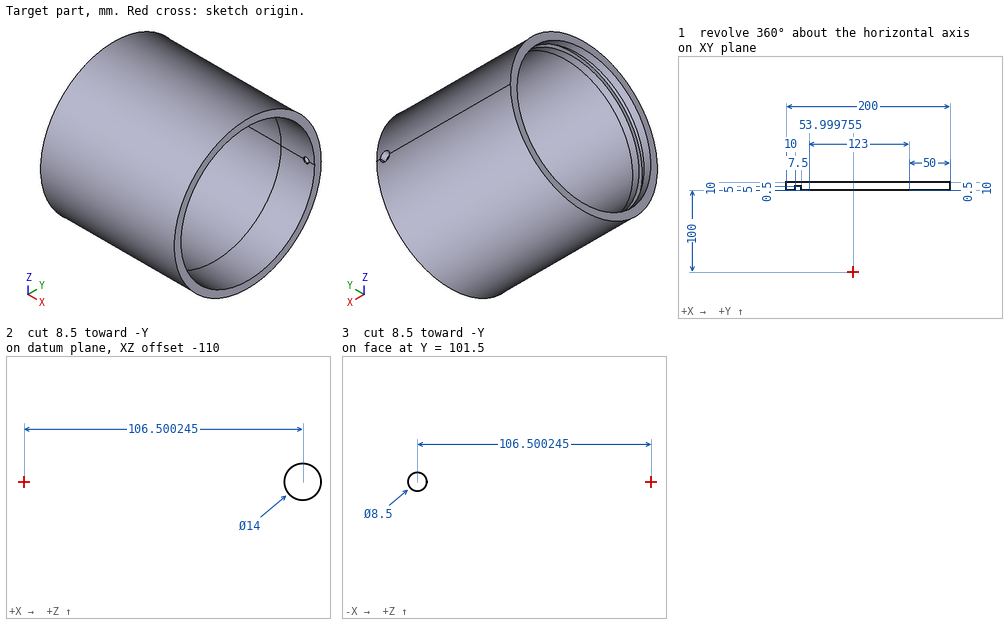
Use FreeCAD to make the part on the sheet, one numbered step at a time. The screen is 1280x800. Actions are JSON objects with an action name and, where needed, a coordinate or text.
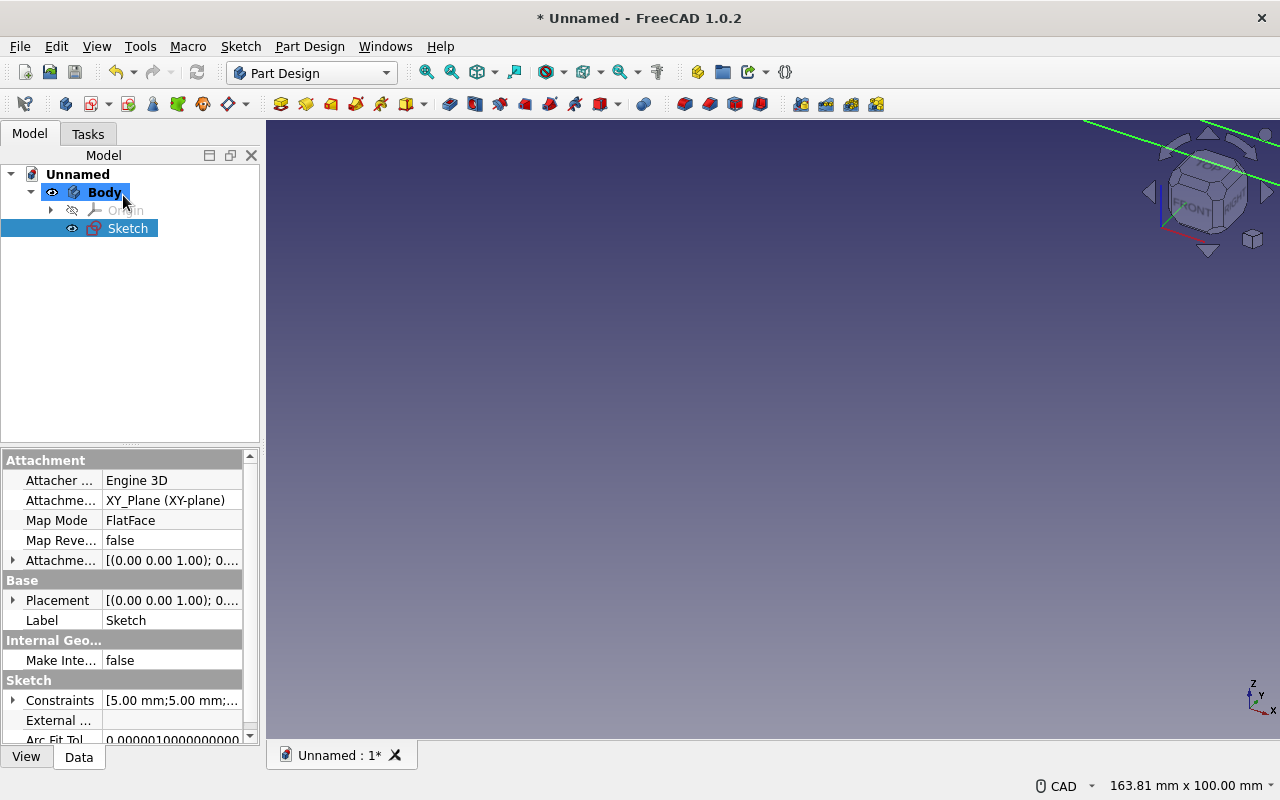
{"action": "left_click", "coordinate": [306, 104]}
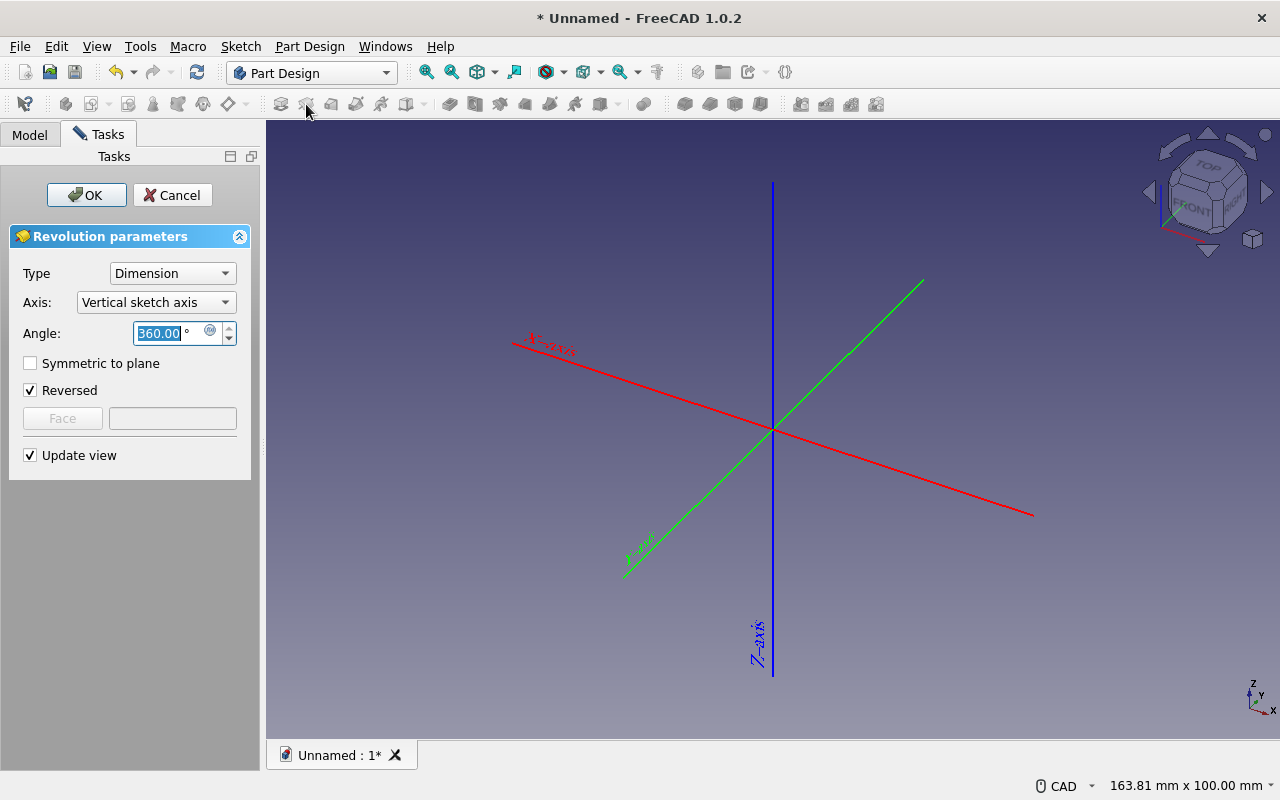
{"action": "left_click", "coordinate": [157, 302]}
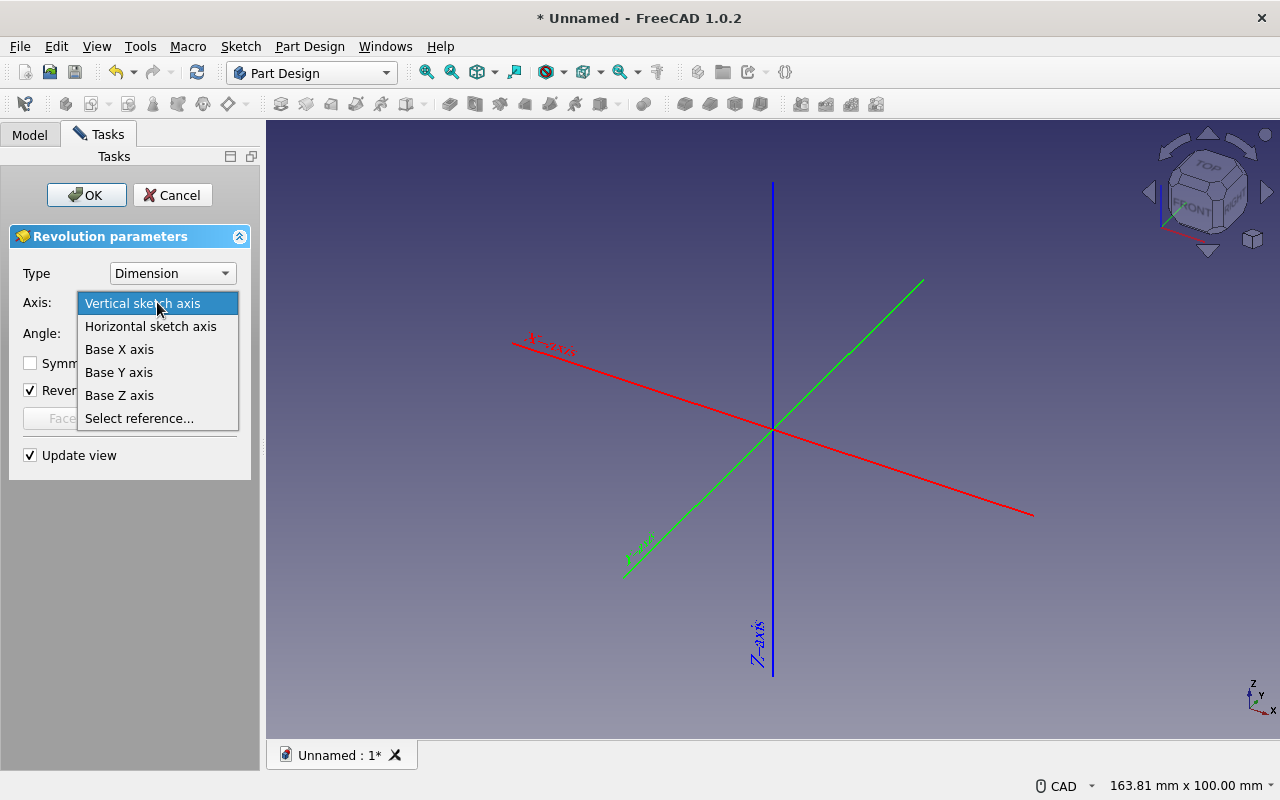
{"action": "left_click", "coordinate": [156, 326]}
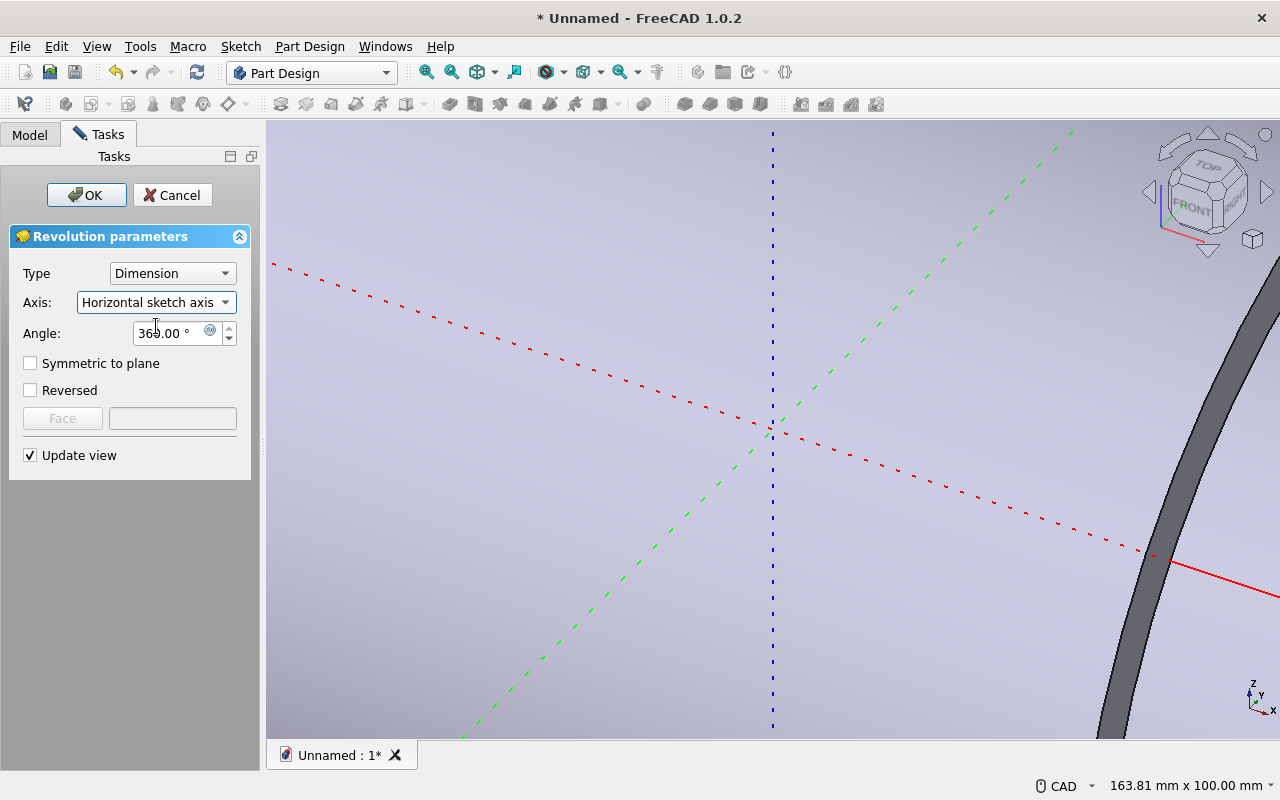
{"action": "left_click", "coordinate": [87, 195]}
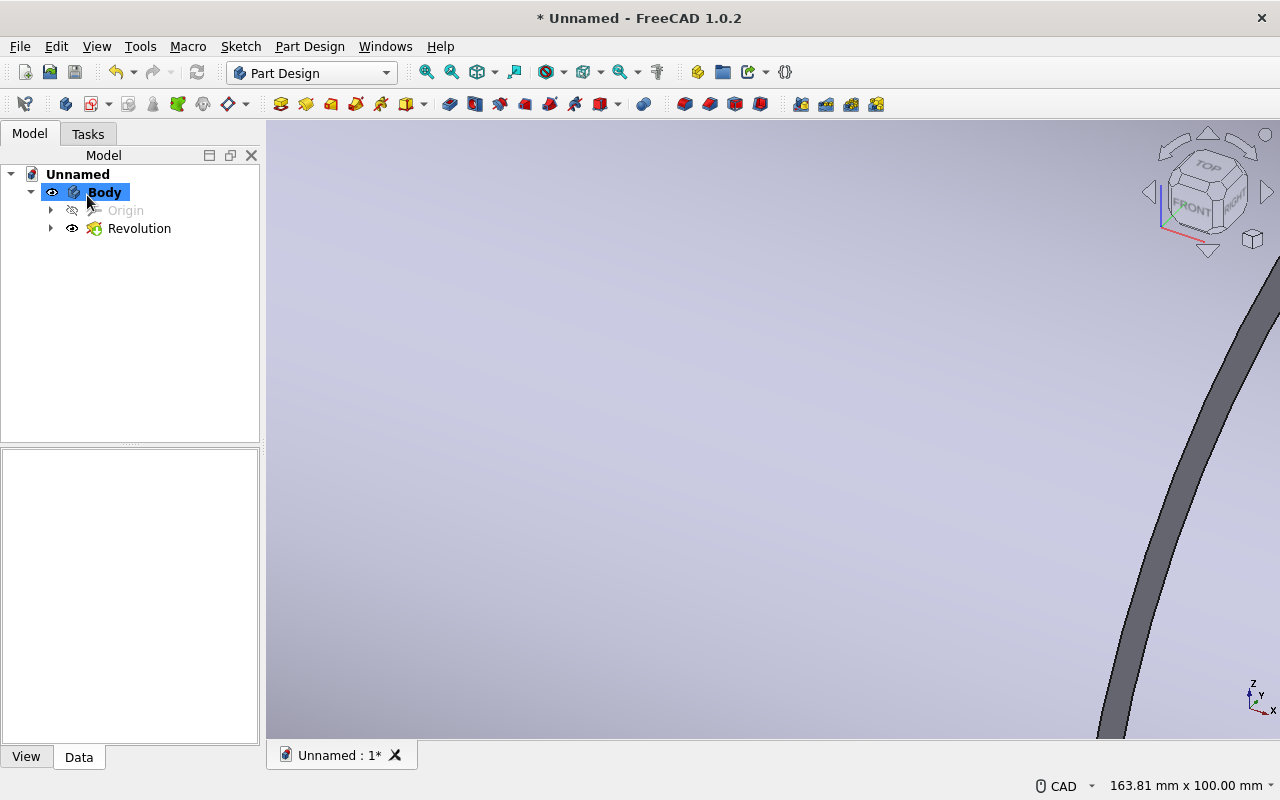
{"action": "left_click", "coordinate": [427, 72]}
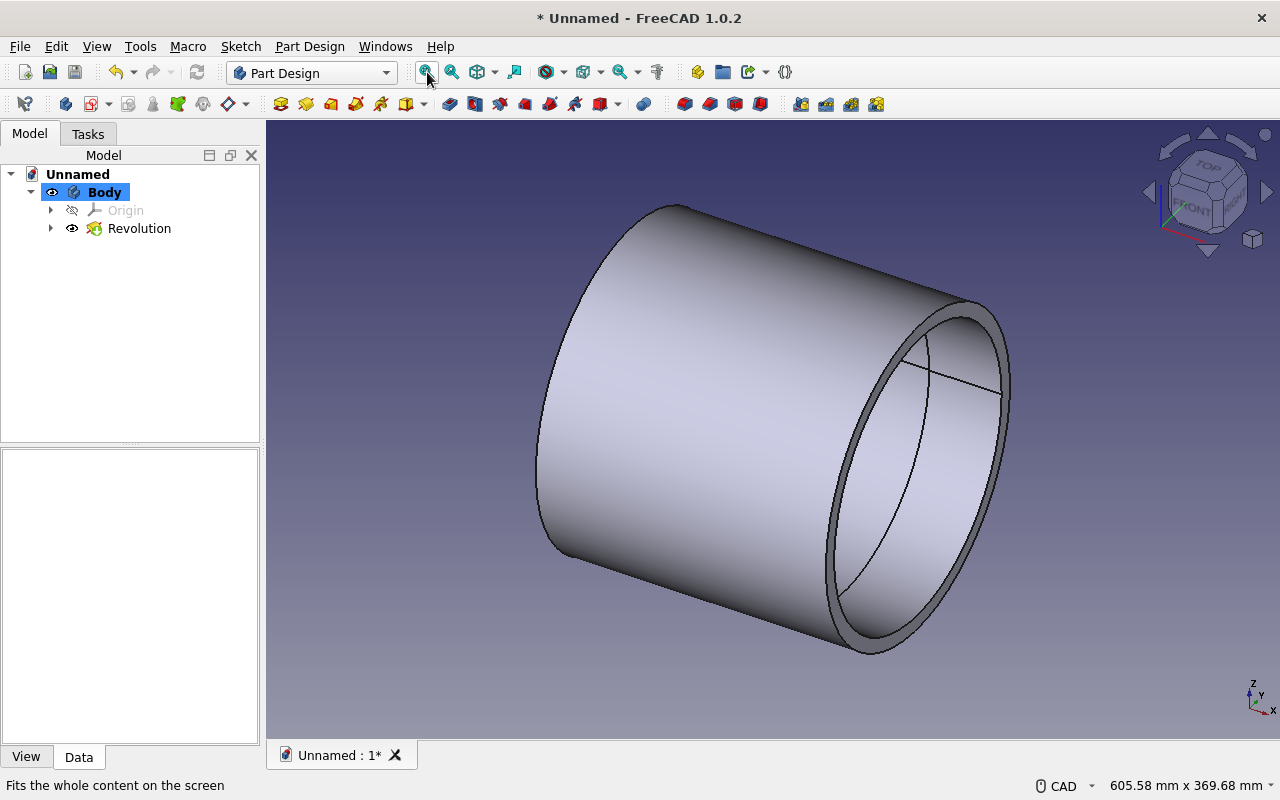
{"action": "left_click", "coordinate": [51, 210]}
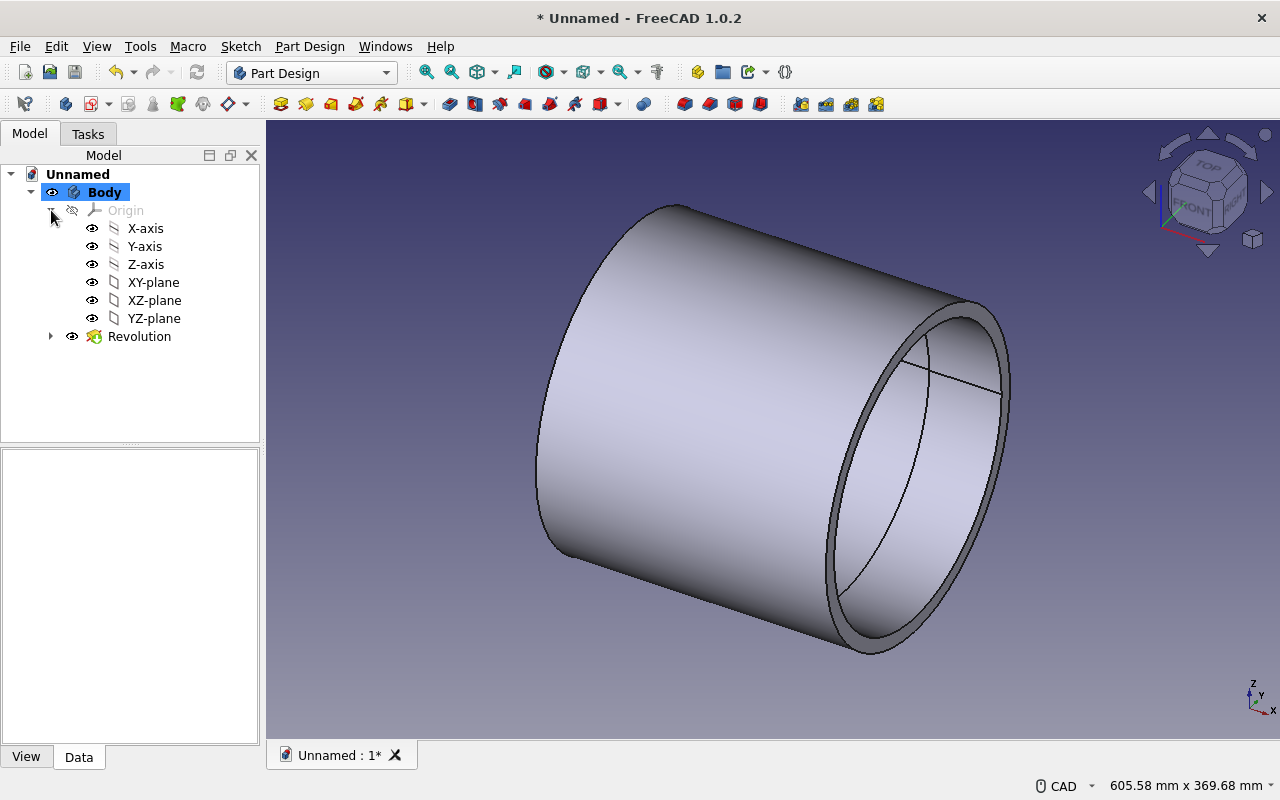
{"action": "left_click", "coordinate": [137, 300]}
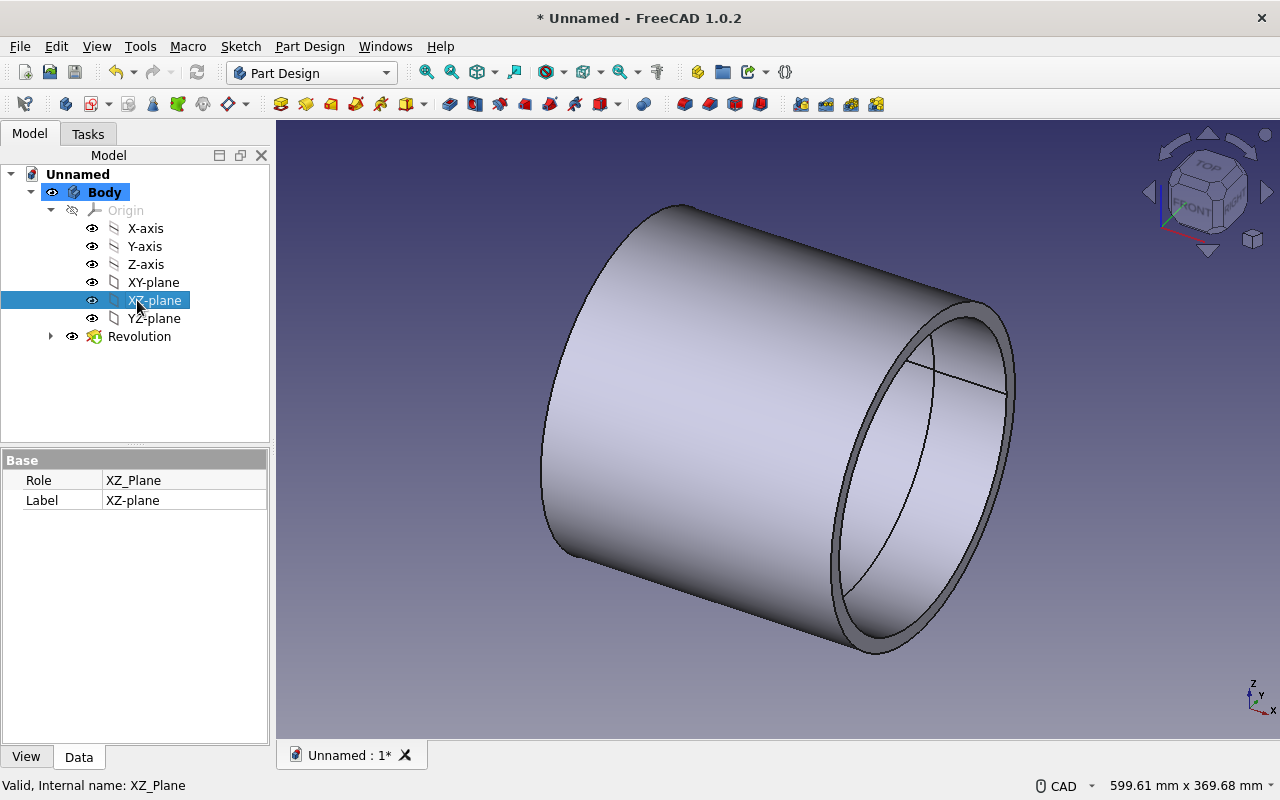
{"action": "left_click", "coordinate": [228, 104]}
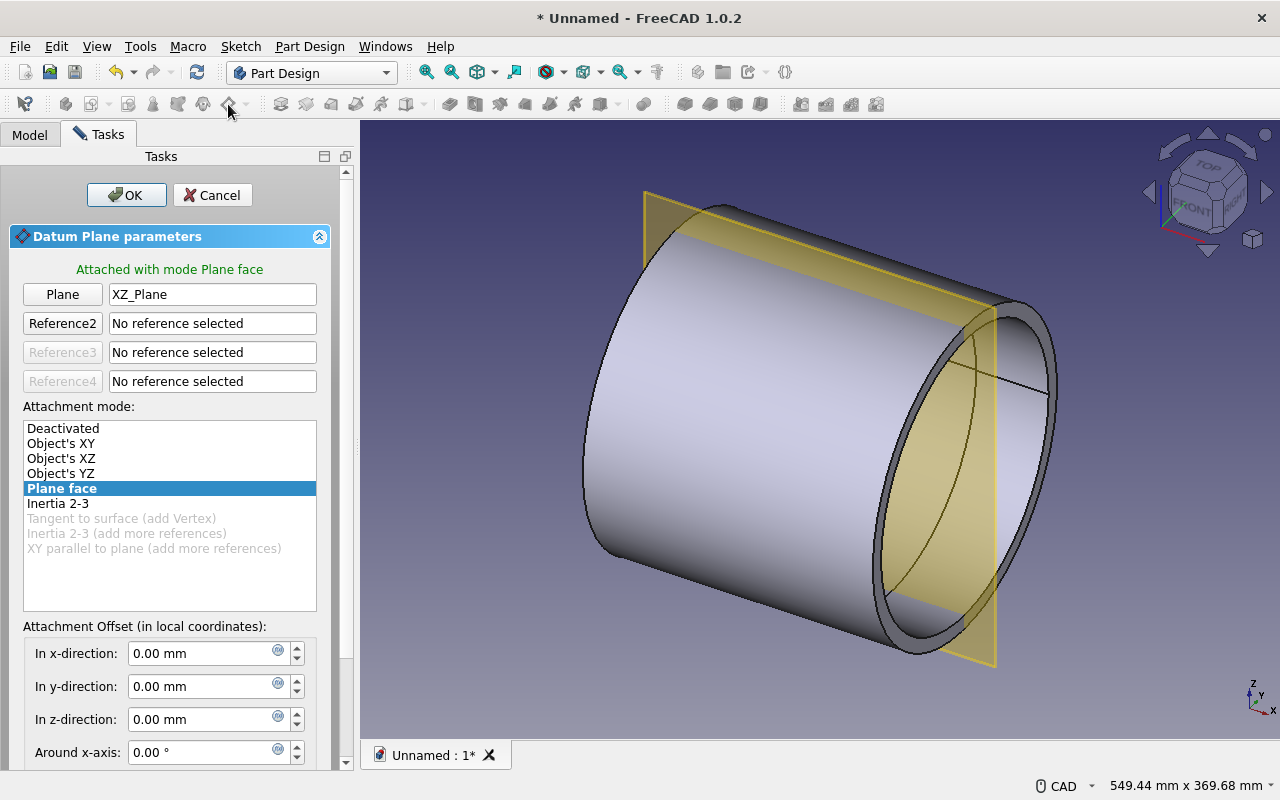
{"action": "triple_click", "coordinate": [210, 720]}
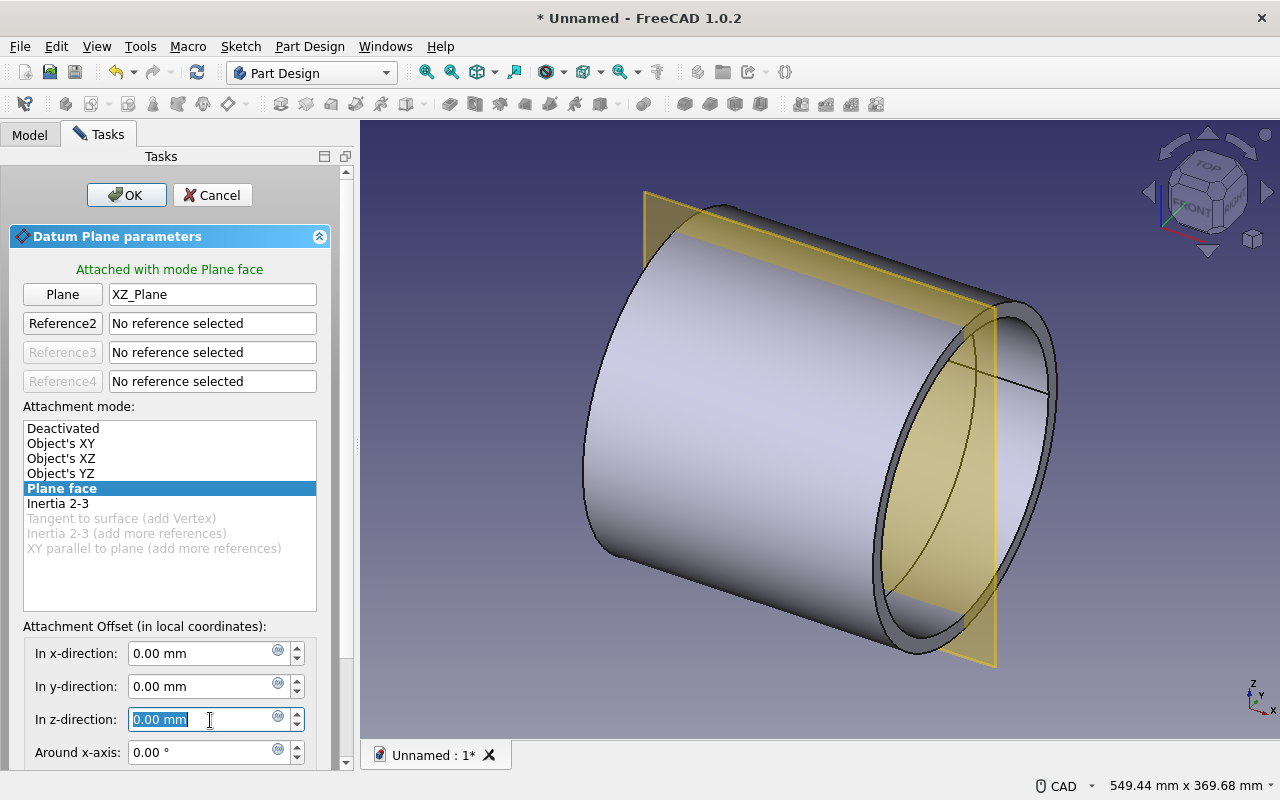
{"action": "type", "text": "-110"}
{"action": "key", "text": "Tab"}